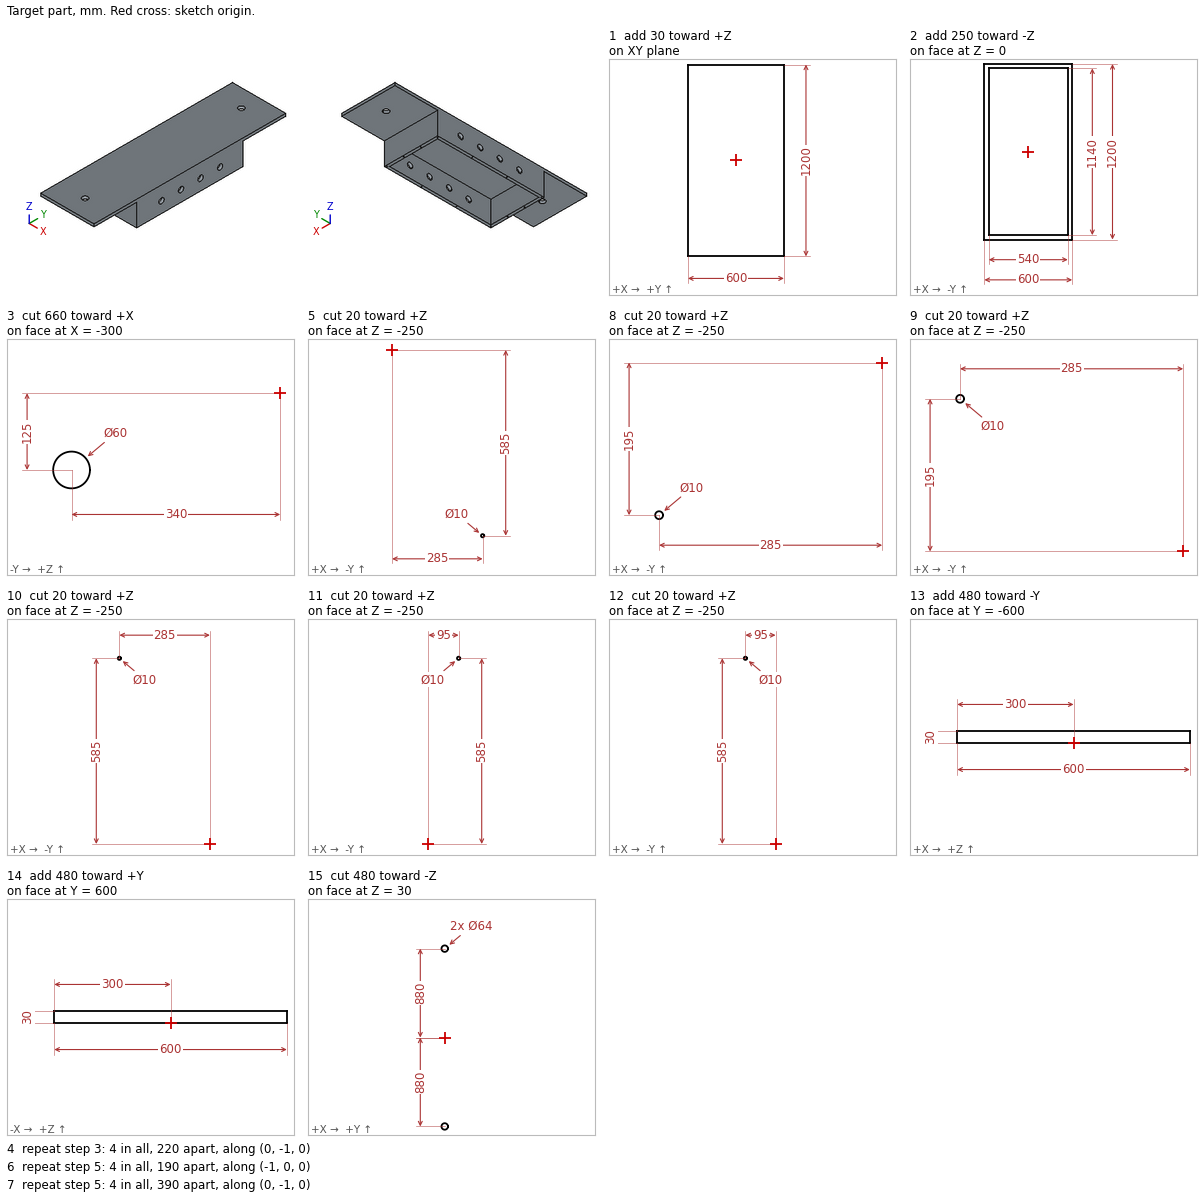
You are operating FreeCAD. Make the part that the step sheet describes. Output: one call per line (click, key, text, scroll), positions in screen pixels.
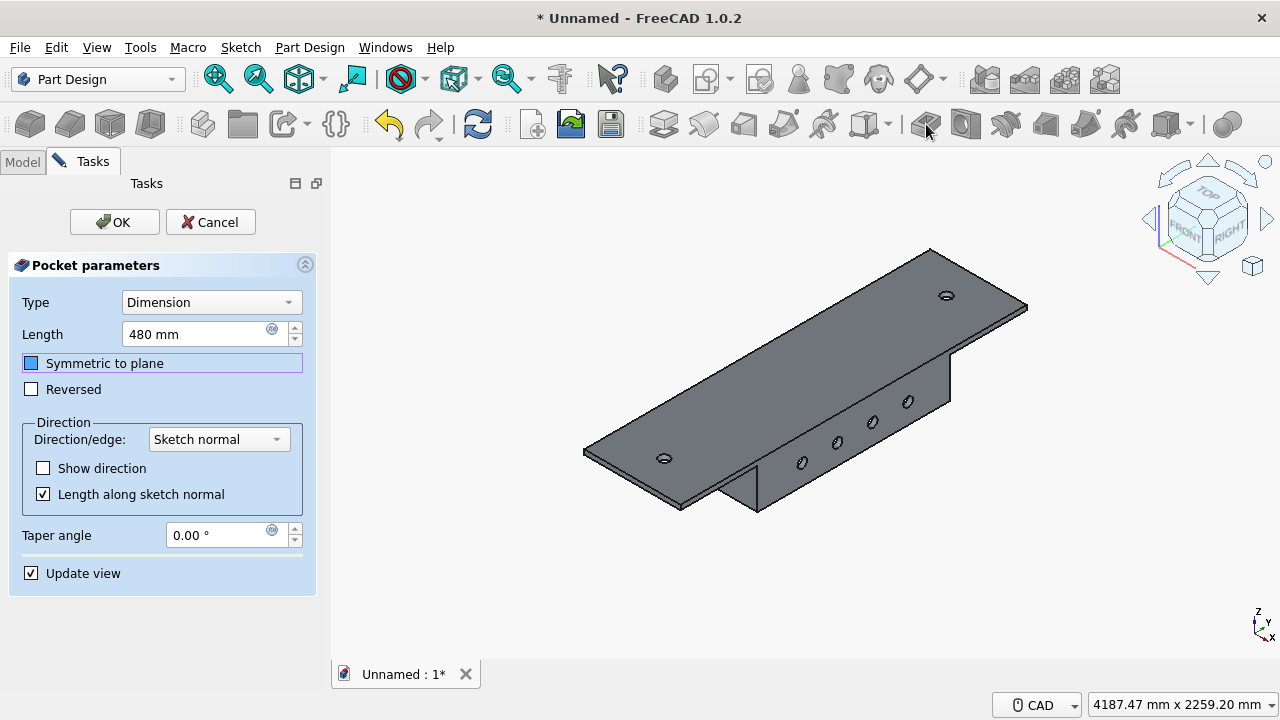
click(115, 222)